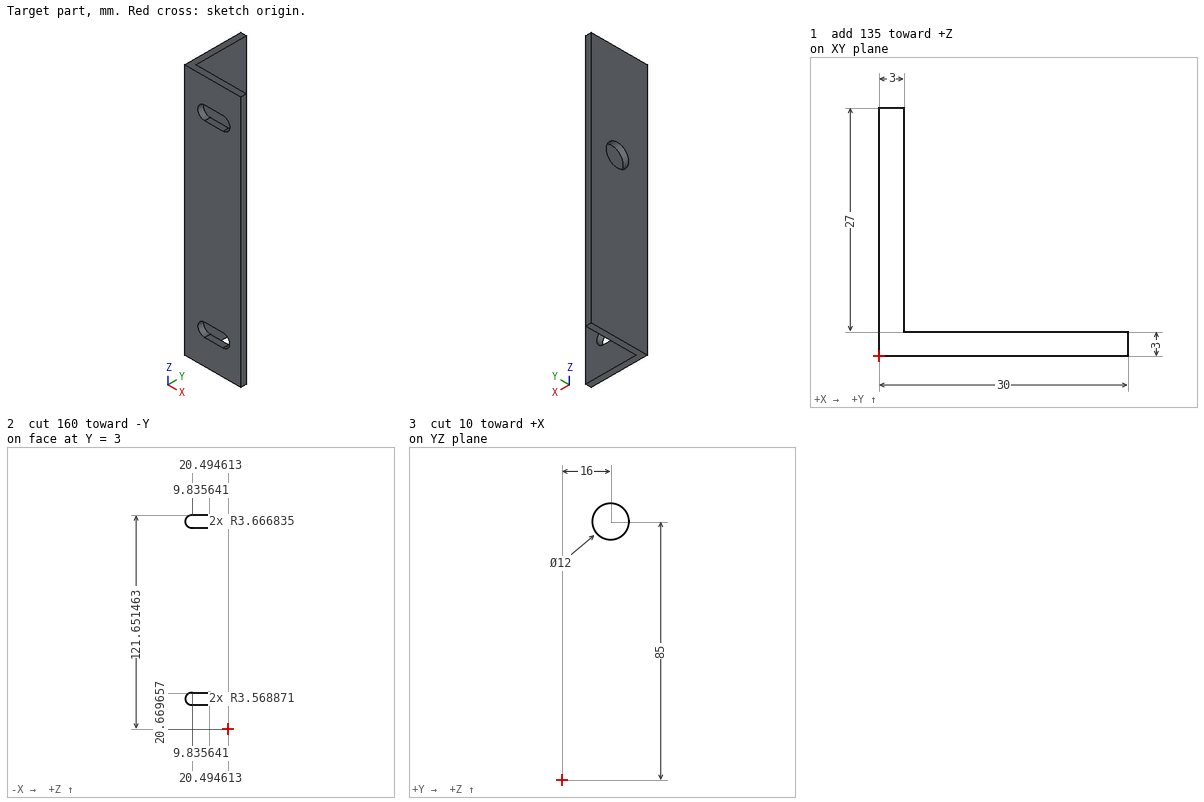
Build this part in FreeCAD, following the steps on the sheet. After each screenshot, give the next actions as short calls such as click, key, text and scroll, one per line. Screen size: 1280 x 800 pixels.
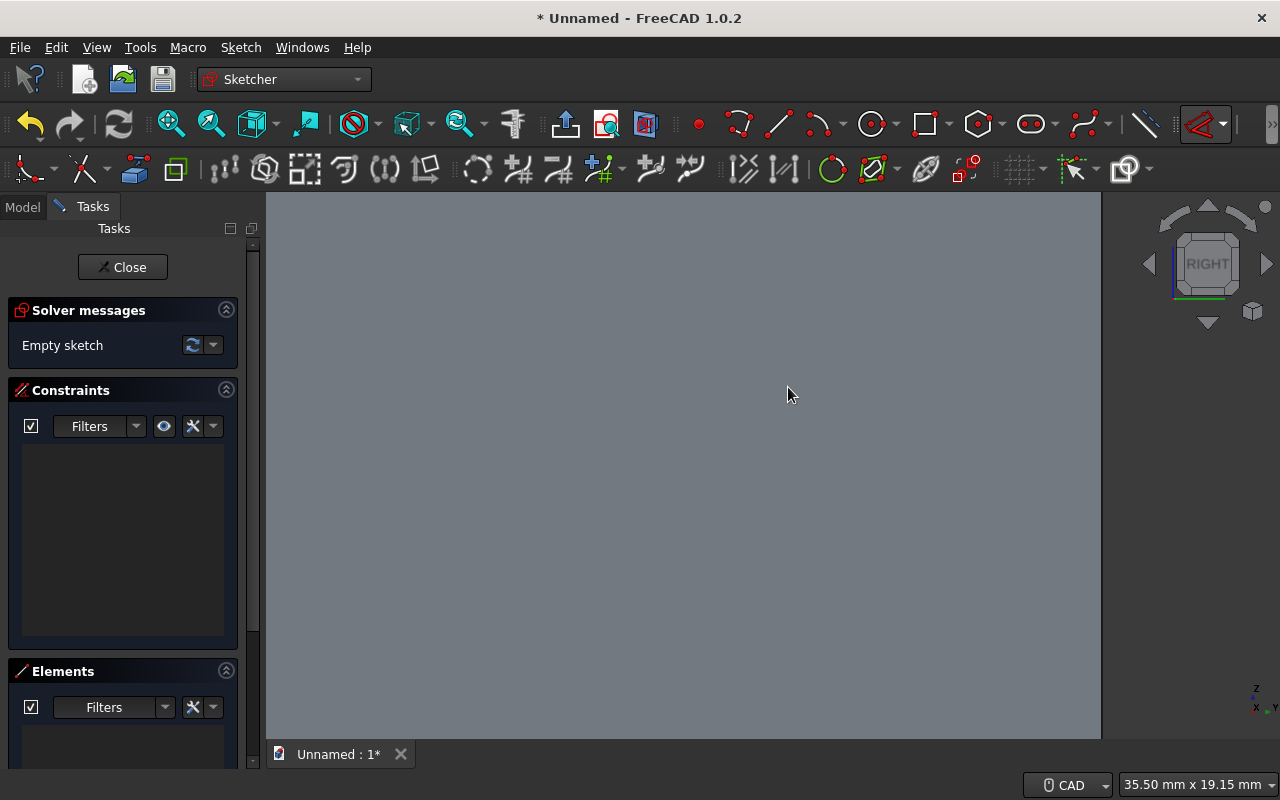
key(g)
key(c)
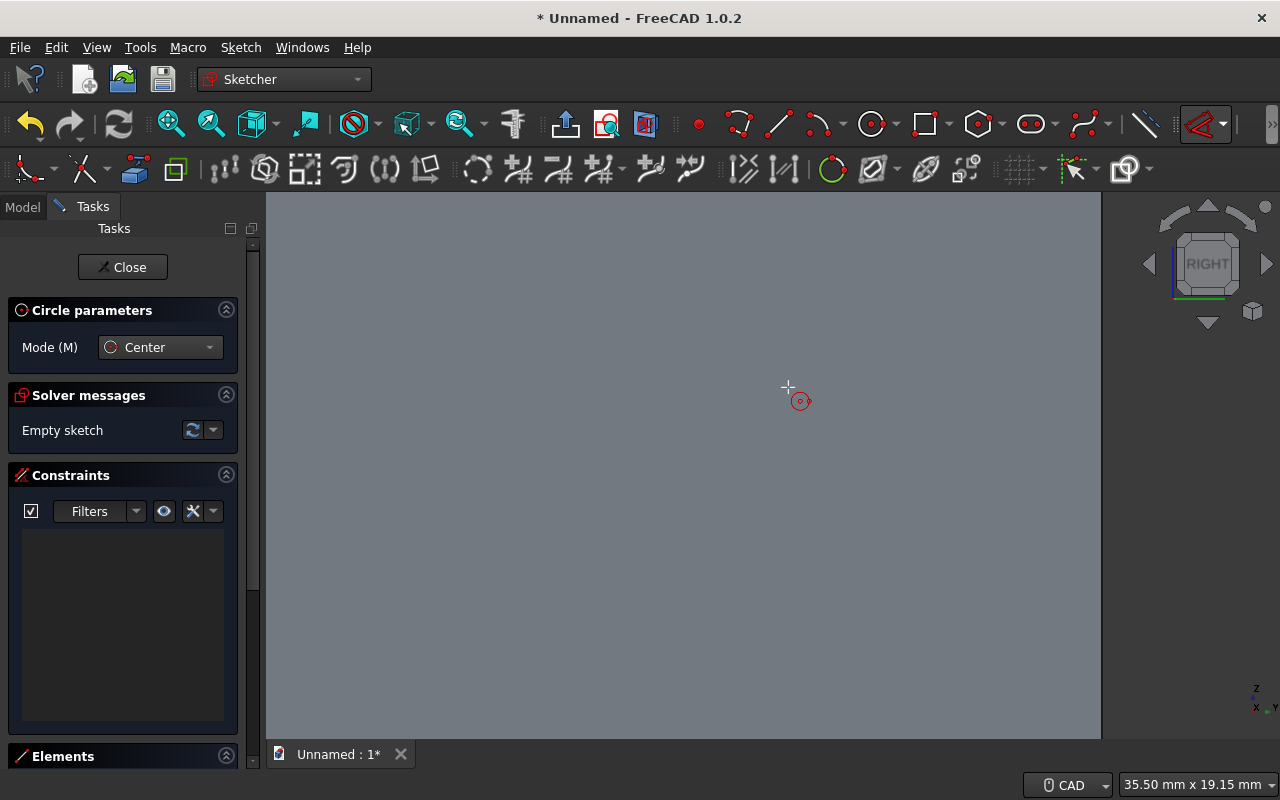
click(702, 465)
click(824, 344)
key(Escape)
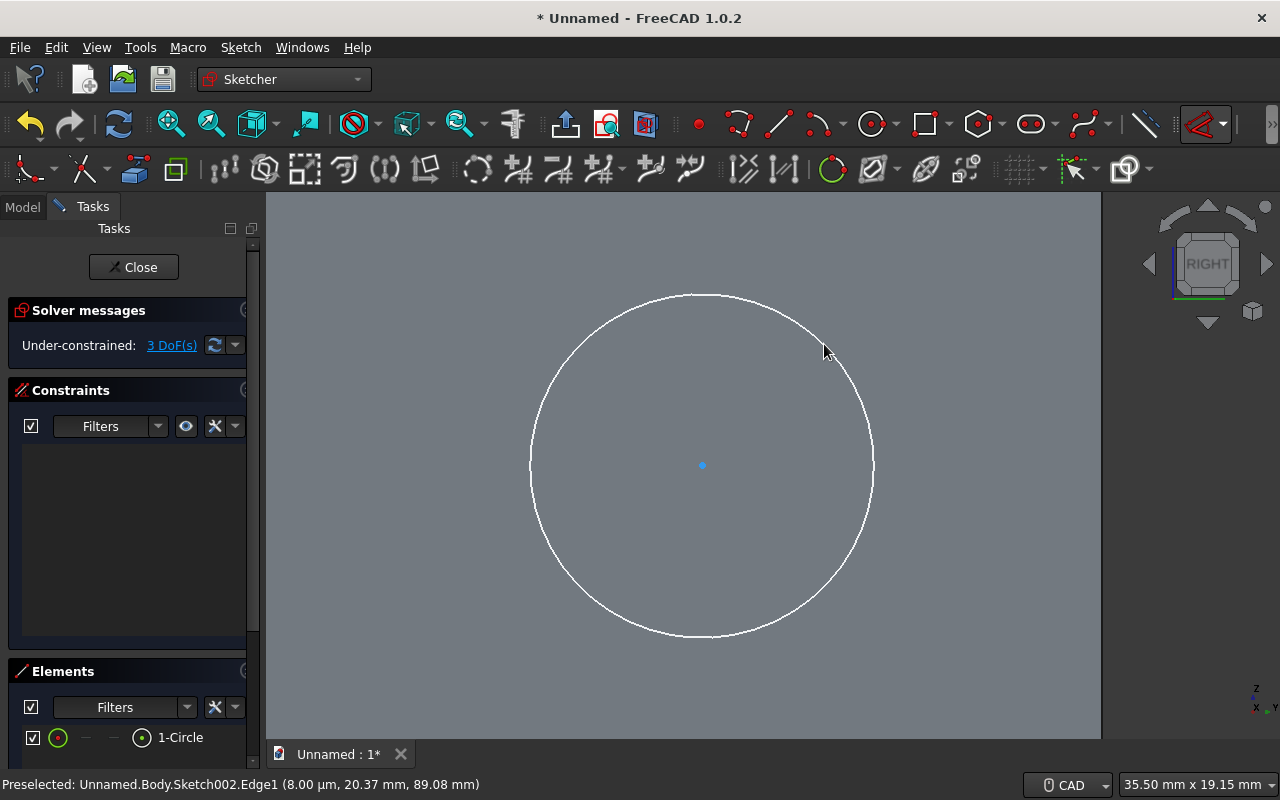
click(823, 344)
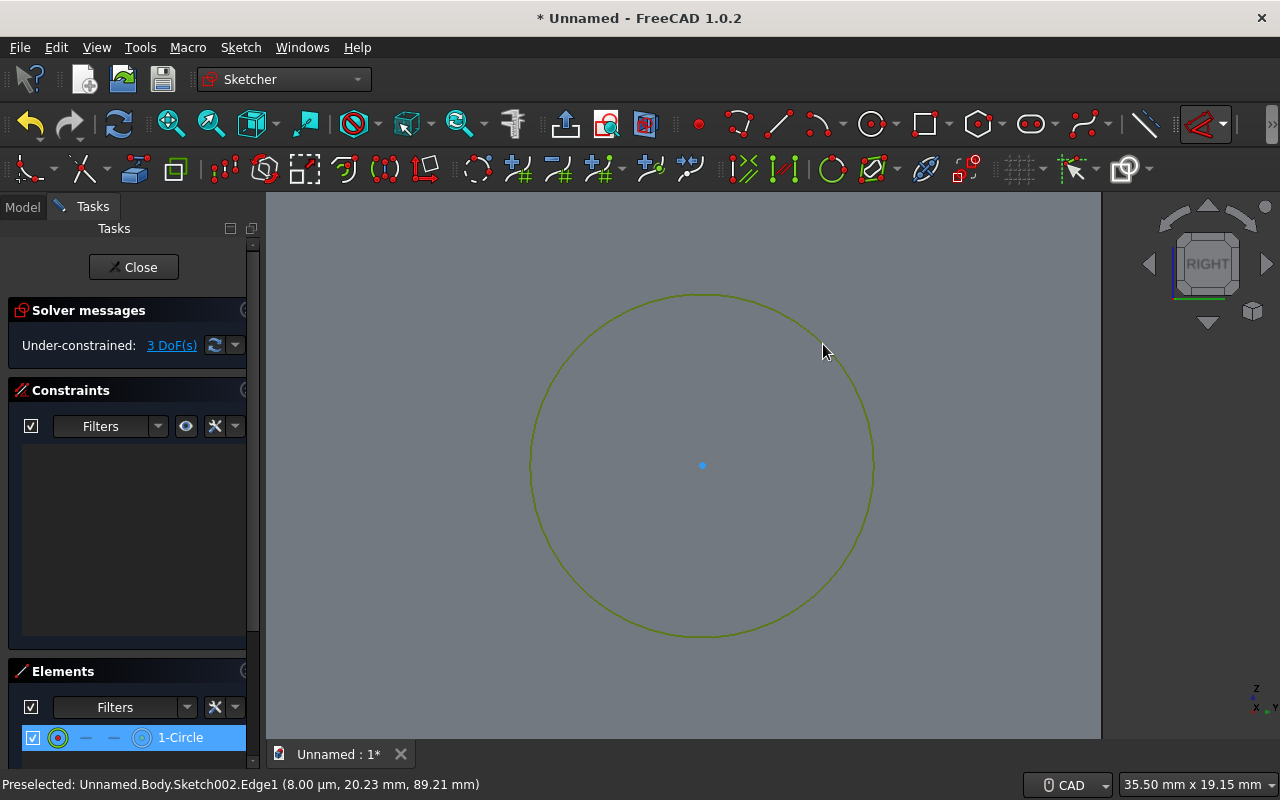
key(k)
key(o)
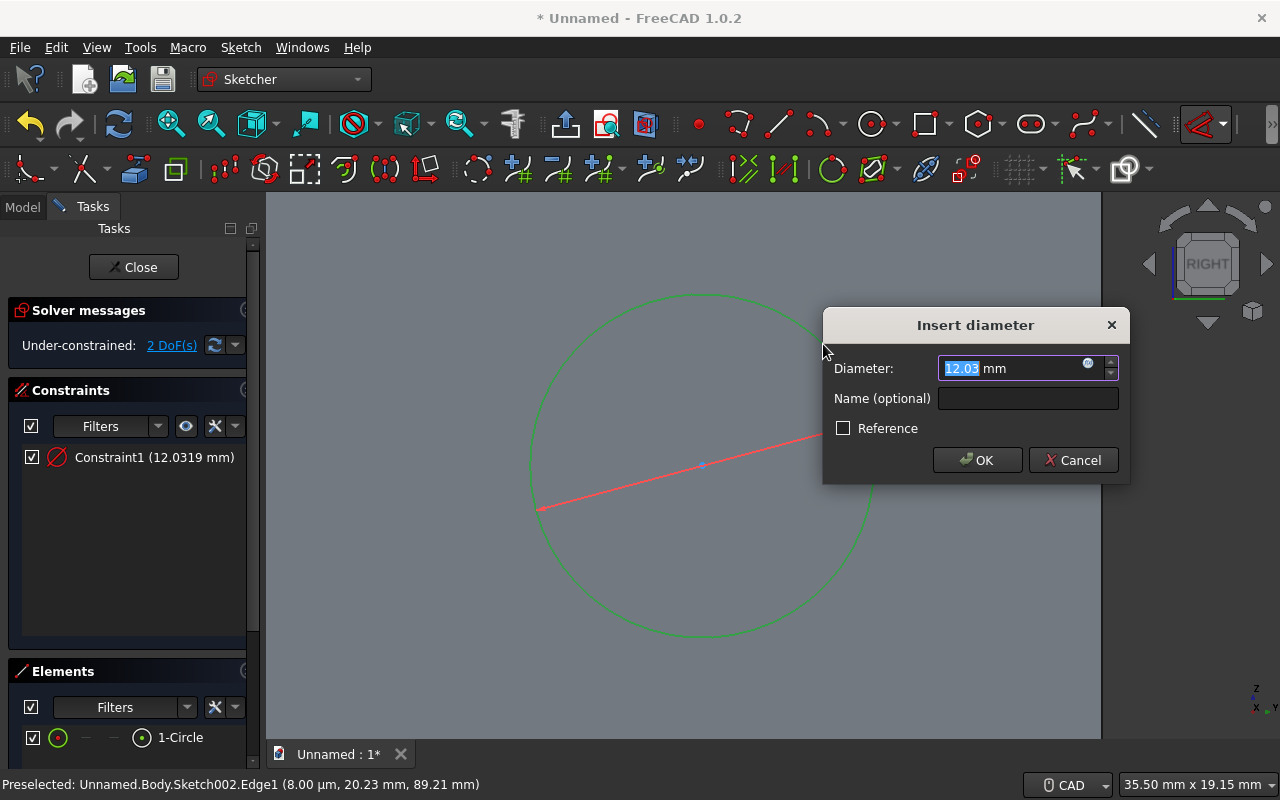
text(12)
key(Return)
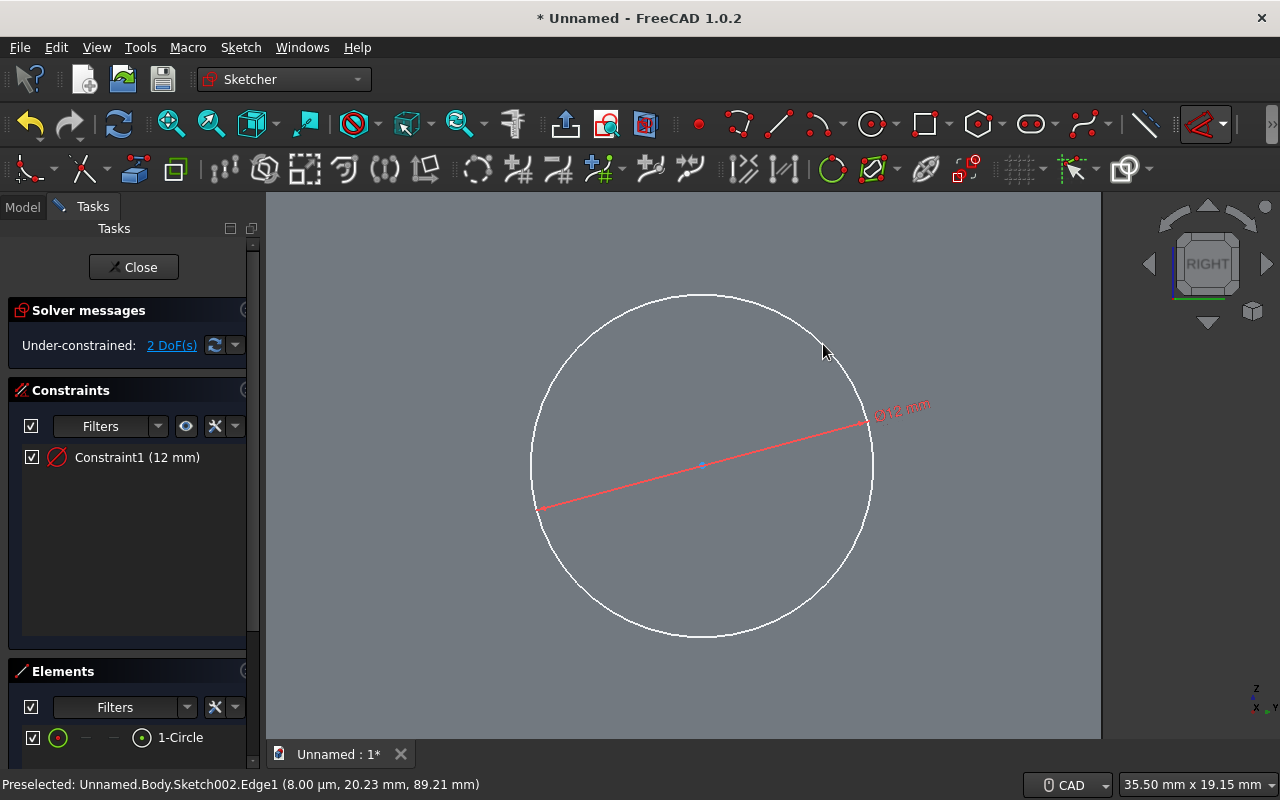
click(702, 466)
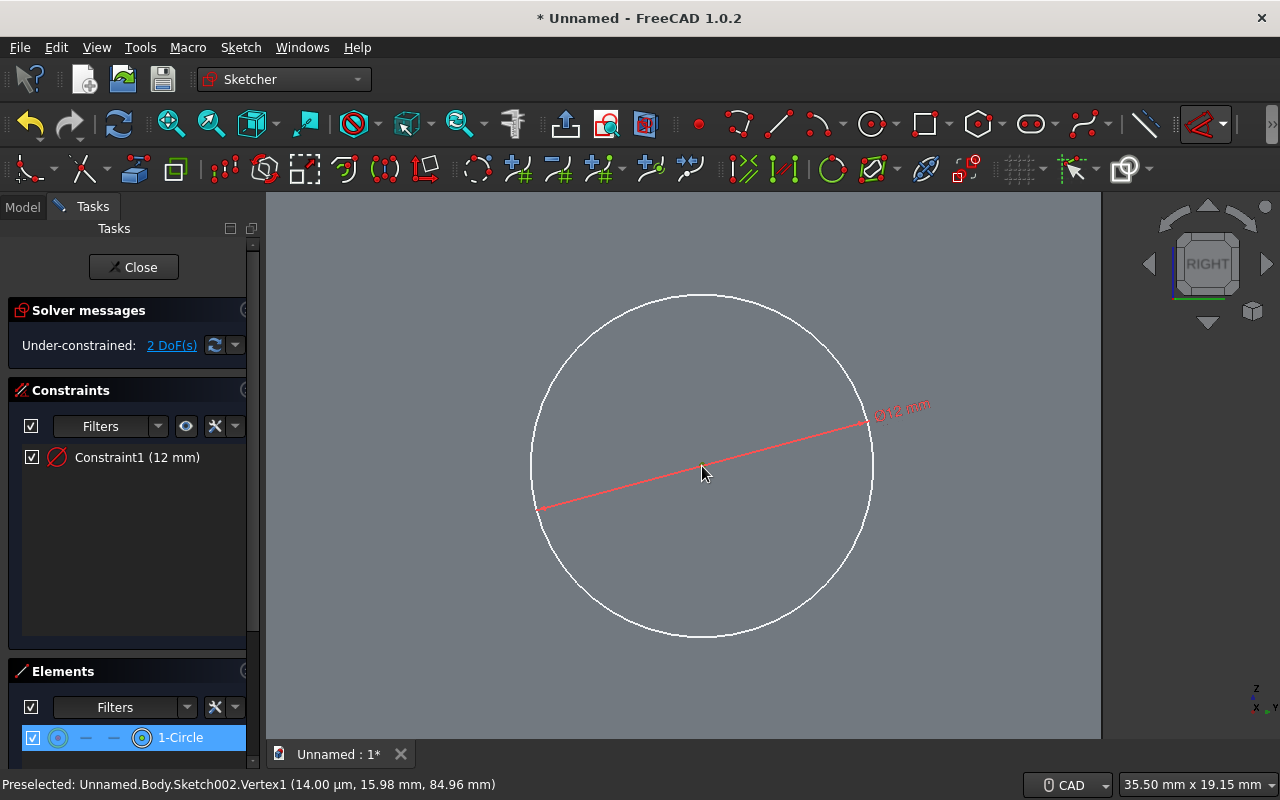
key(l)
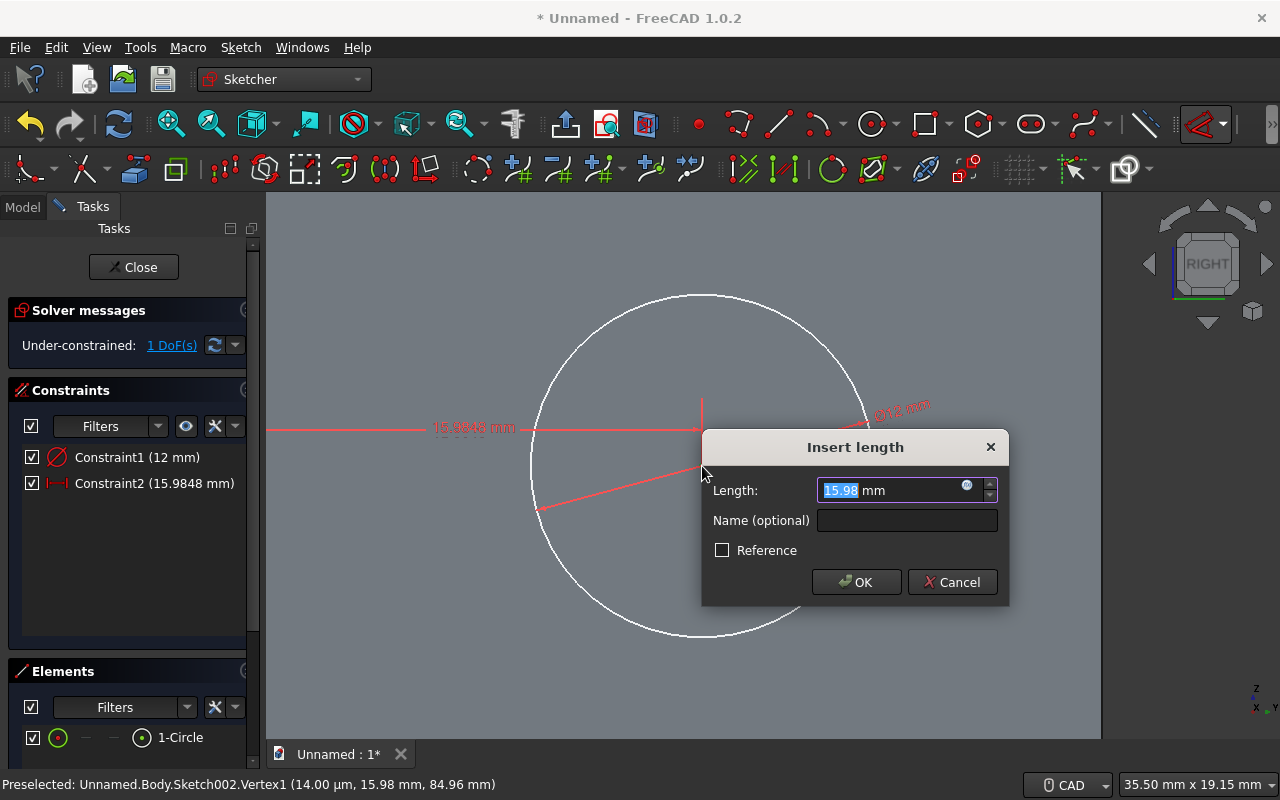
text(16)
key(Return)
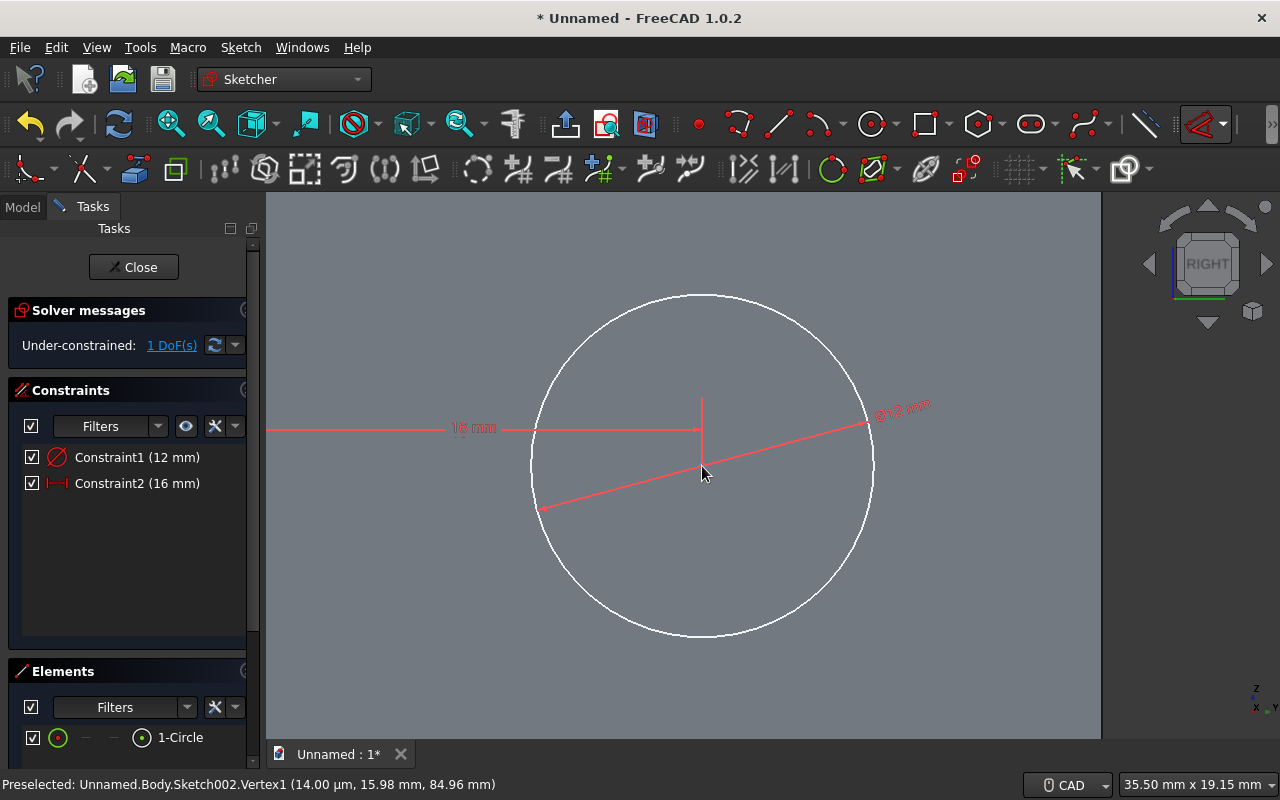
click(702, 466)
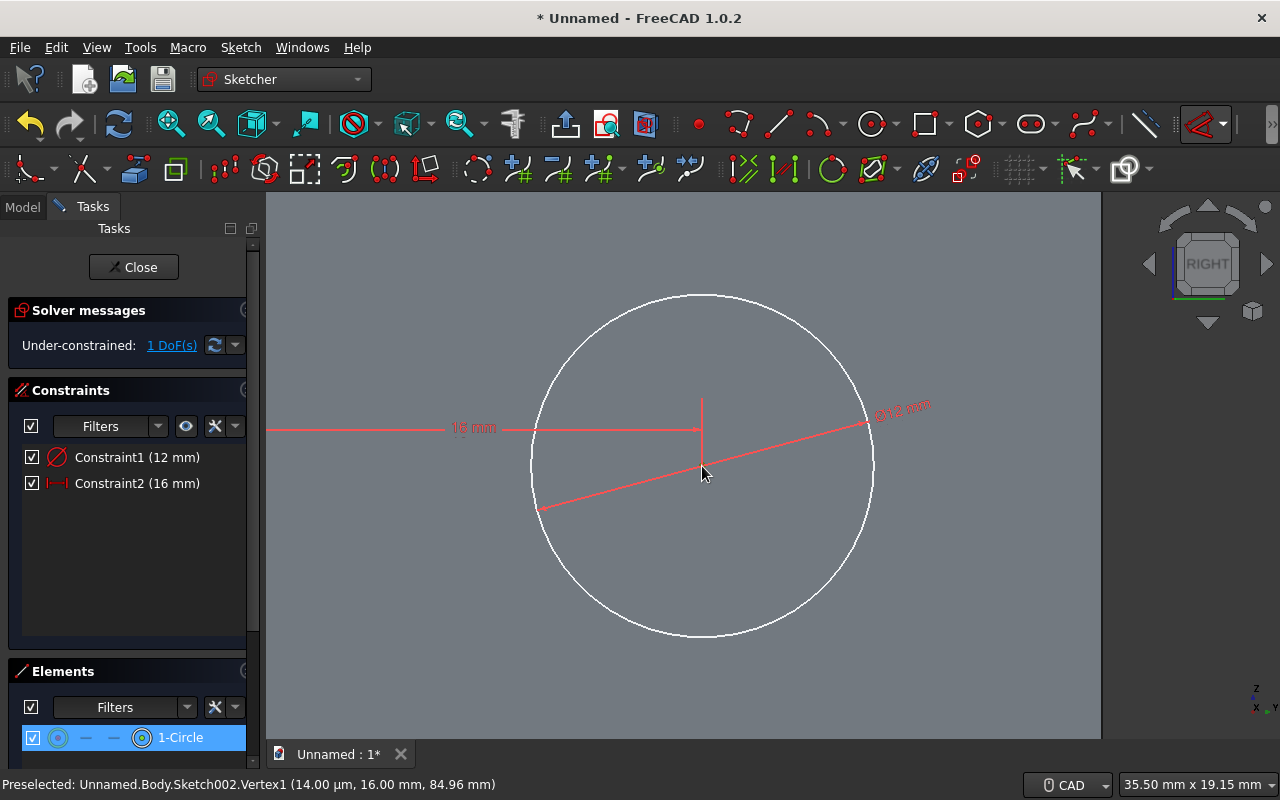
key(i)